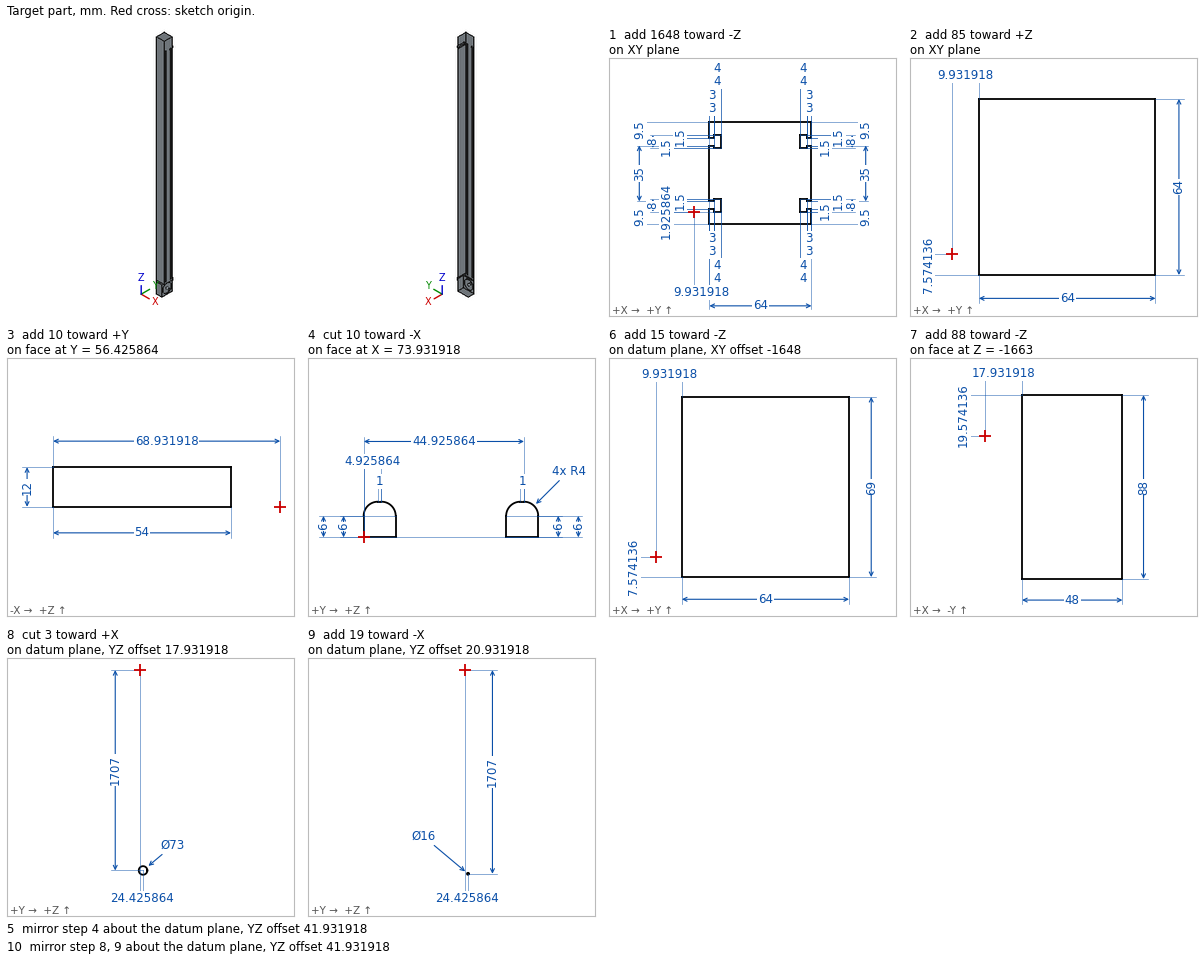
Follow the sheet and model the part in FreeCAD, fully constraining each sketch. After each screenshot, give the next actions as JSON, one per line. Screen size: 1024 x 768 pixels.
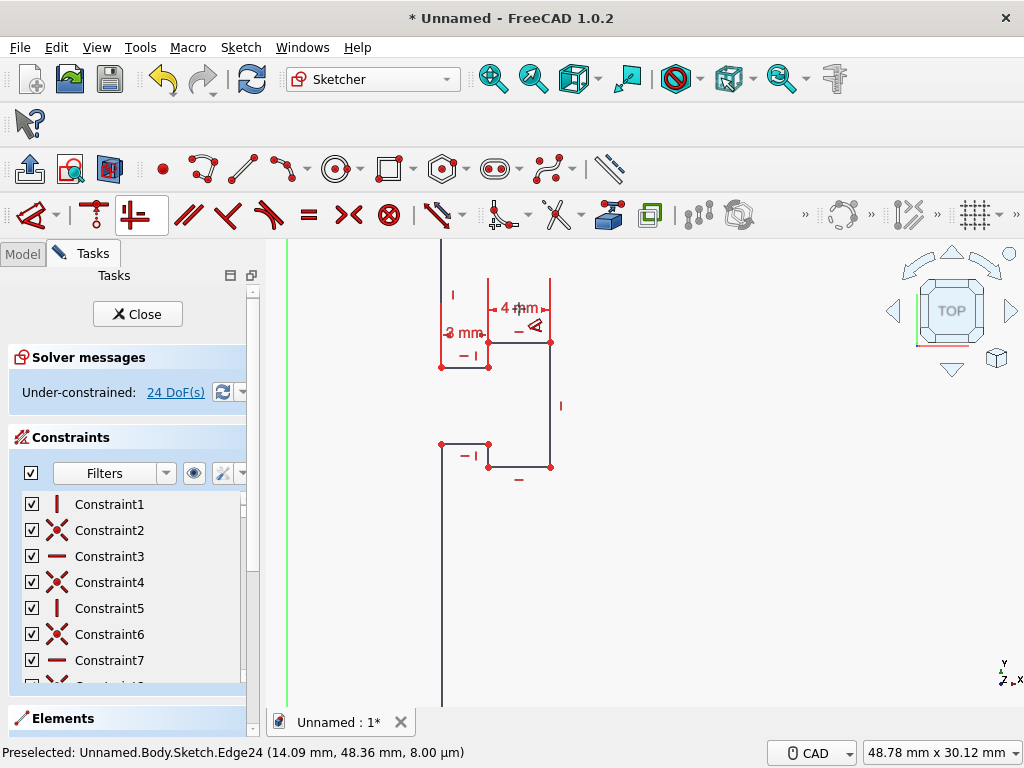
{"action": "left_click", "coordinate": [550, 380]}
{"action": "left_click", "coordinate": [516, 405]}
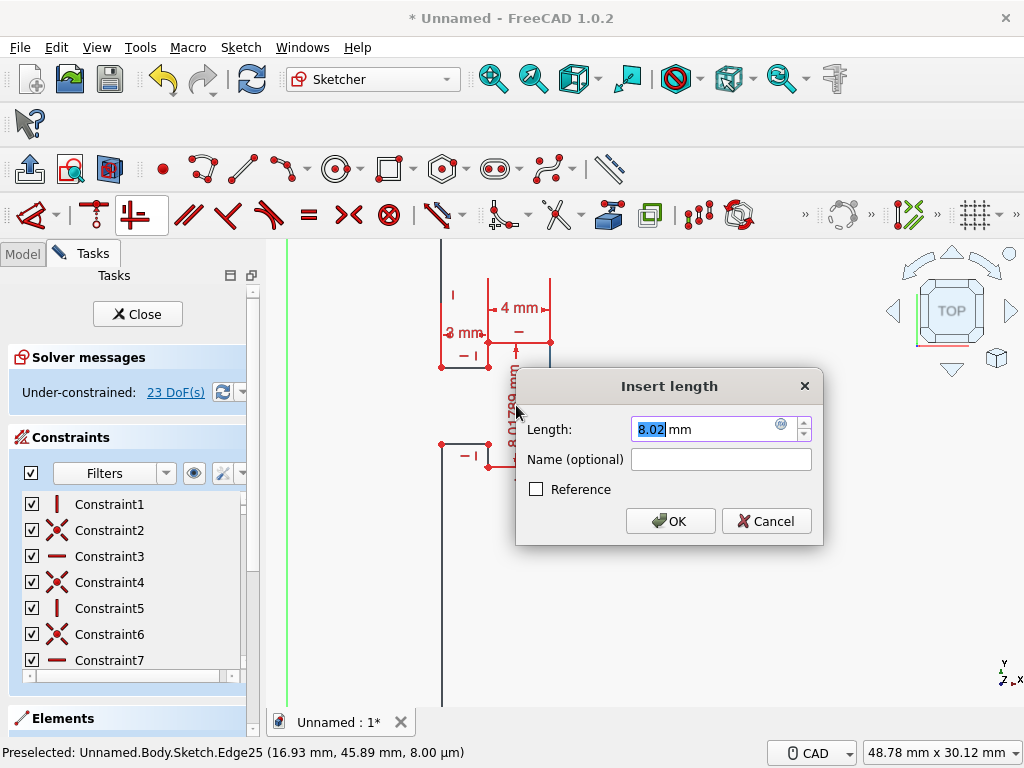
{"action": "type", "text": "8"}
{"action": "key", "text": "Return"}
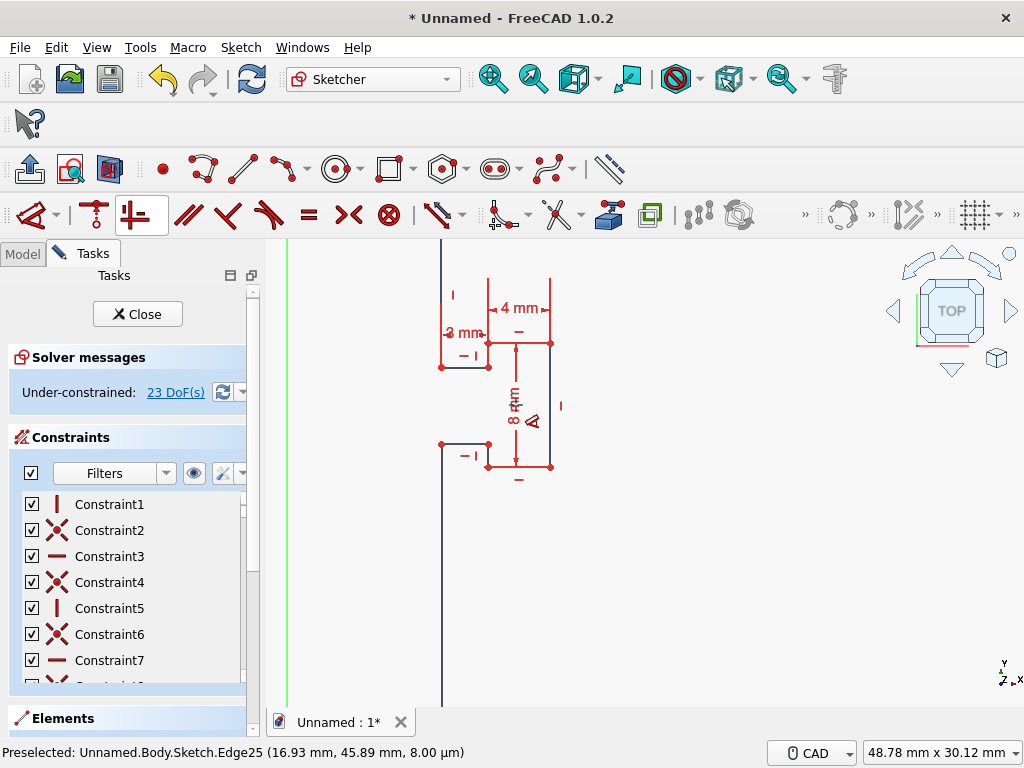
{"action": "left_click", "coordinate": [532, 467]}
{"action": "left_click", "coordinate": [519, 433]}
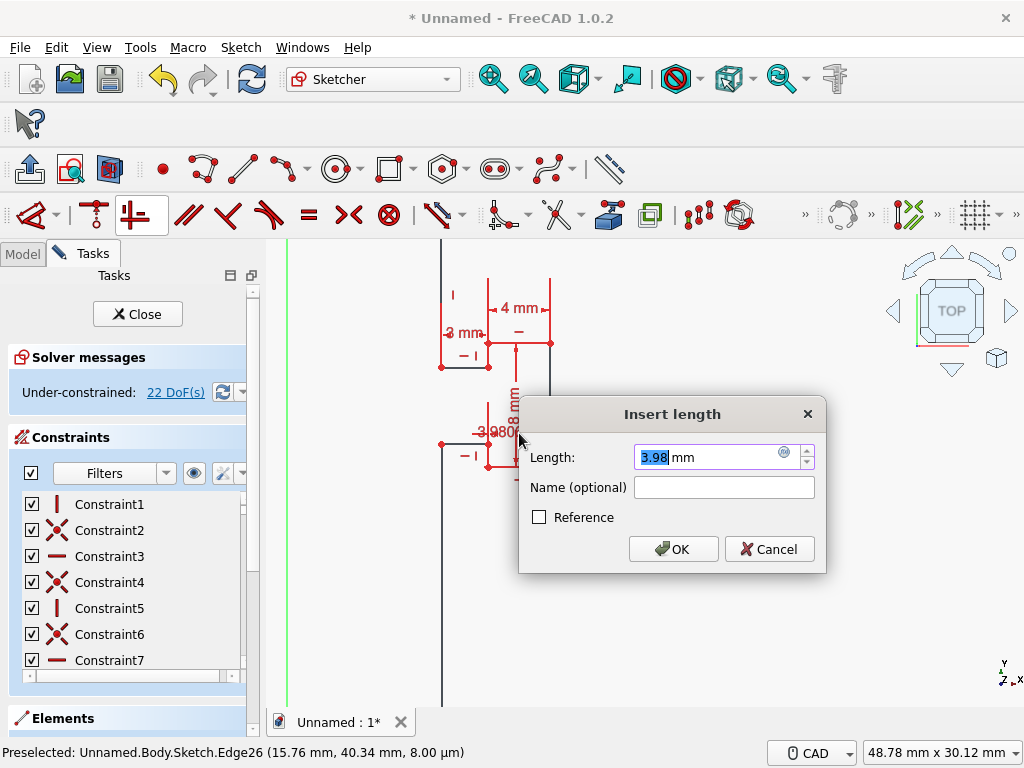
{"action": "type", "text": "4"}
{"action": "key", "text": "Return"}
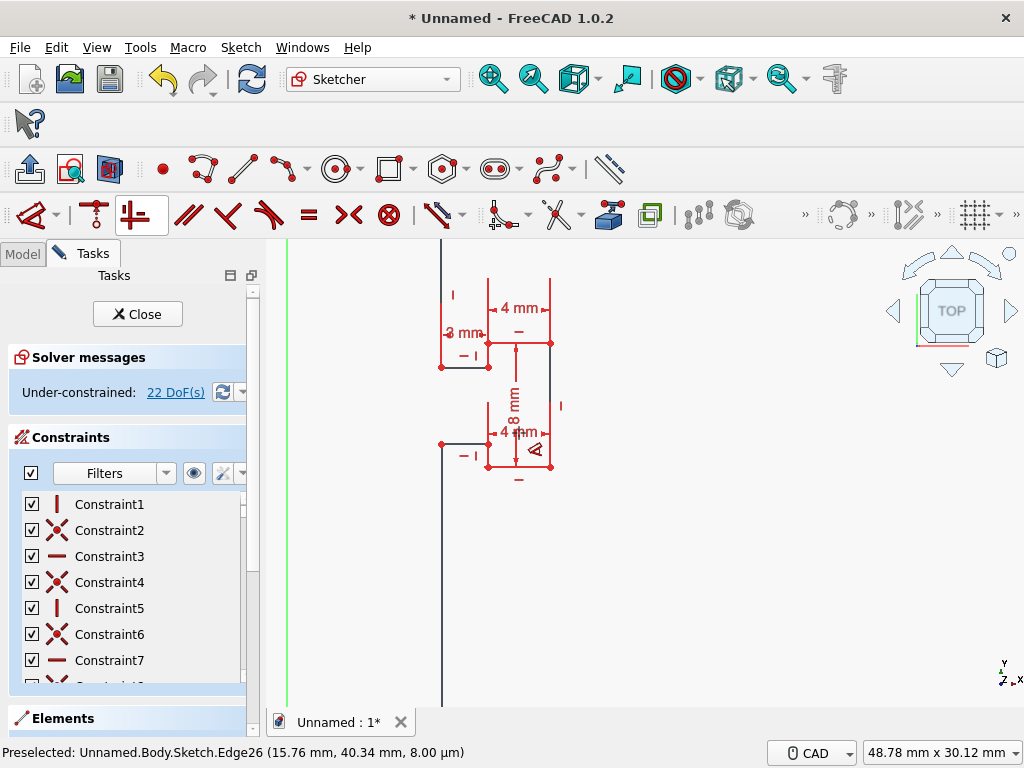
{"action": "left_click", "coordinate": [474, 444]}
{"action": "left_click", "coordinate": [465, 478]}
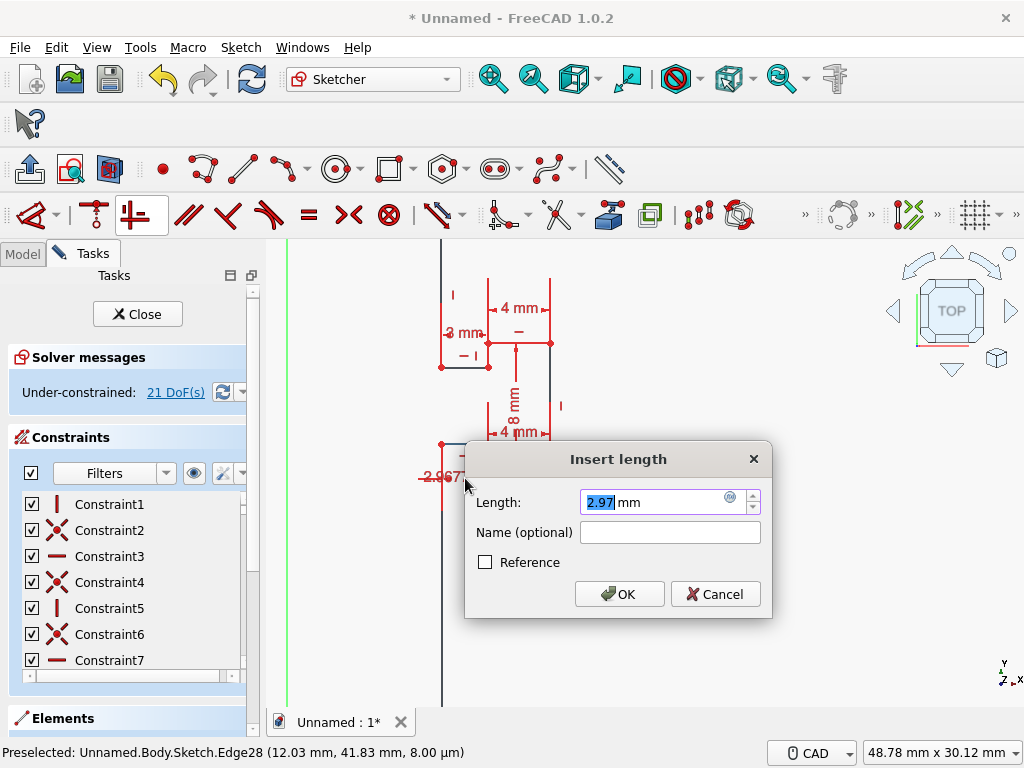
{"action": "type", "text": "3"}
{"action": "key", "text": "Return"}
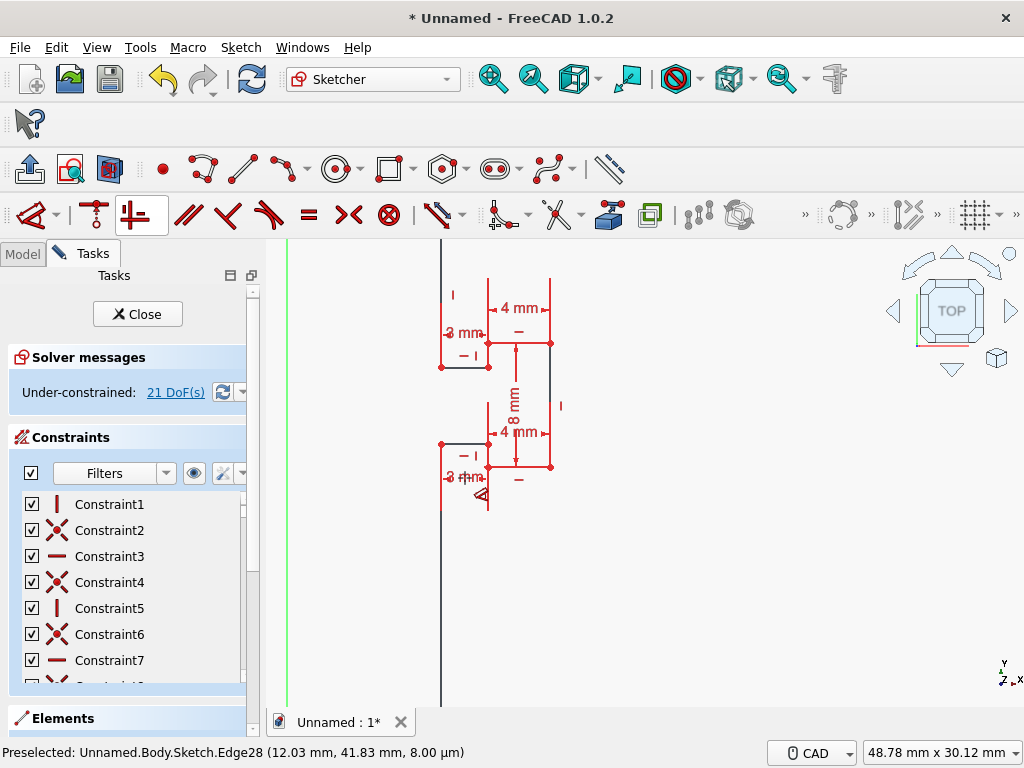
{"action": "scroll", "coordinate": [454, 369], "scroll_direction": "down", "scroll_amount": 6}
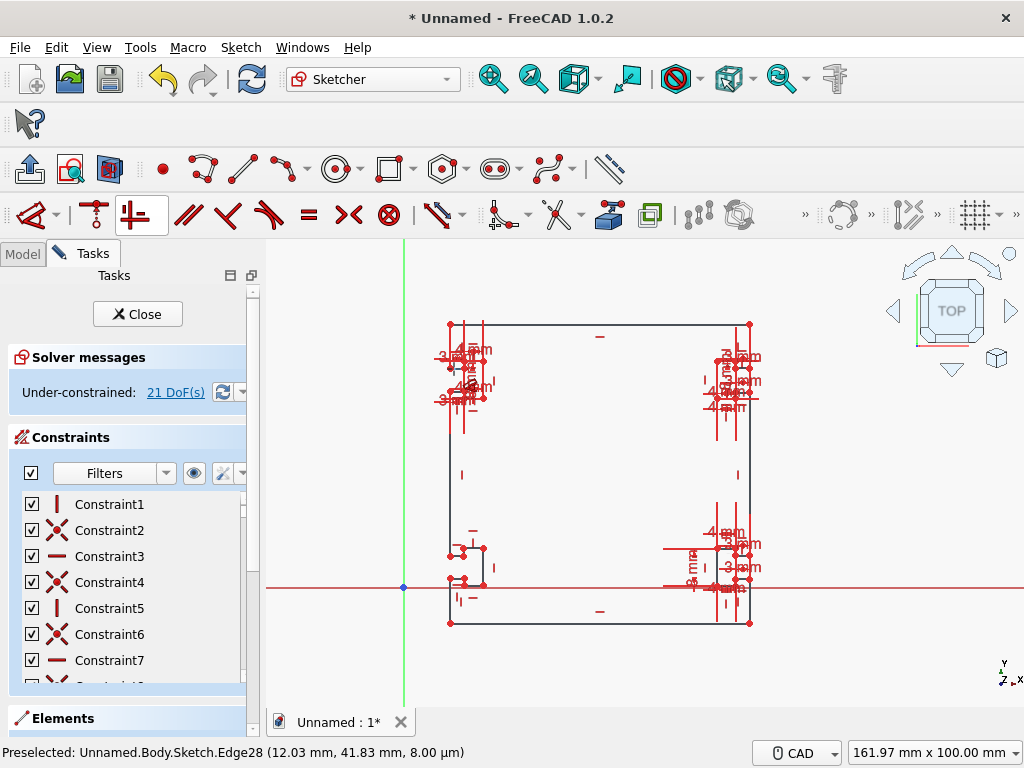
{"action": "scroll", "coordinate": [454, 556], "scroll_direction": "up", "scroll_amount": 7}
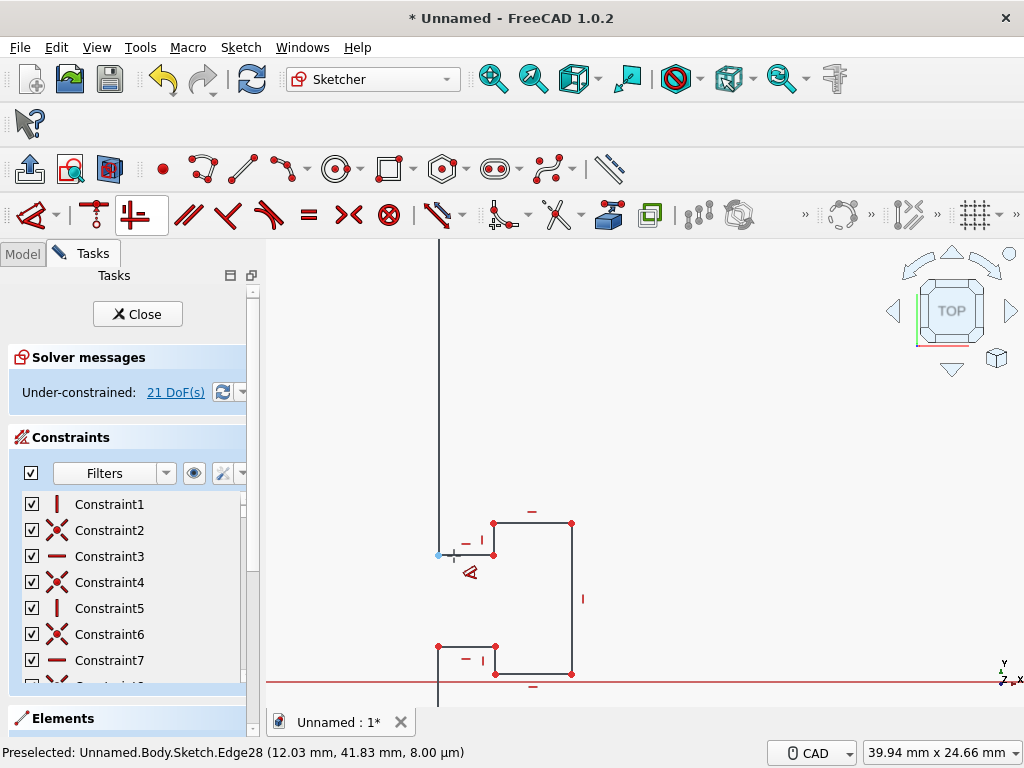
{"action": "left_click", "coordinate": [455, 555]}
{"action": "left_click", "coordinate": [466, 589]}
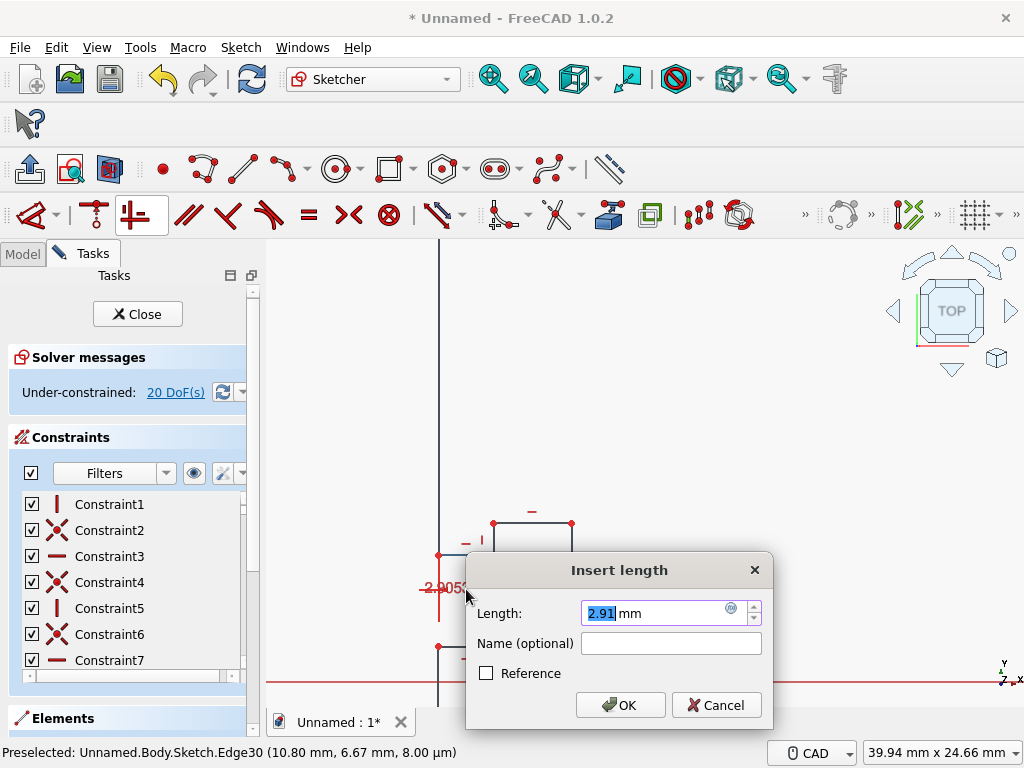
{"action": "type", "text": "3"}
{"action": "key", "text": "Return"}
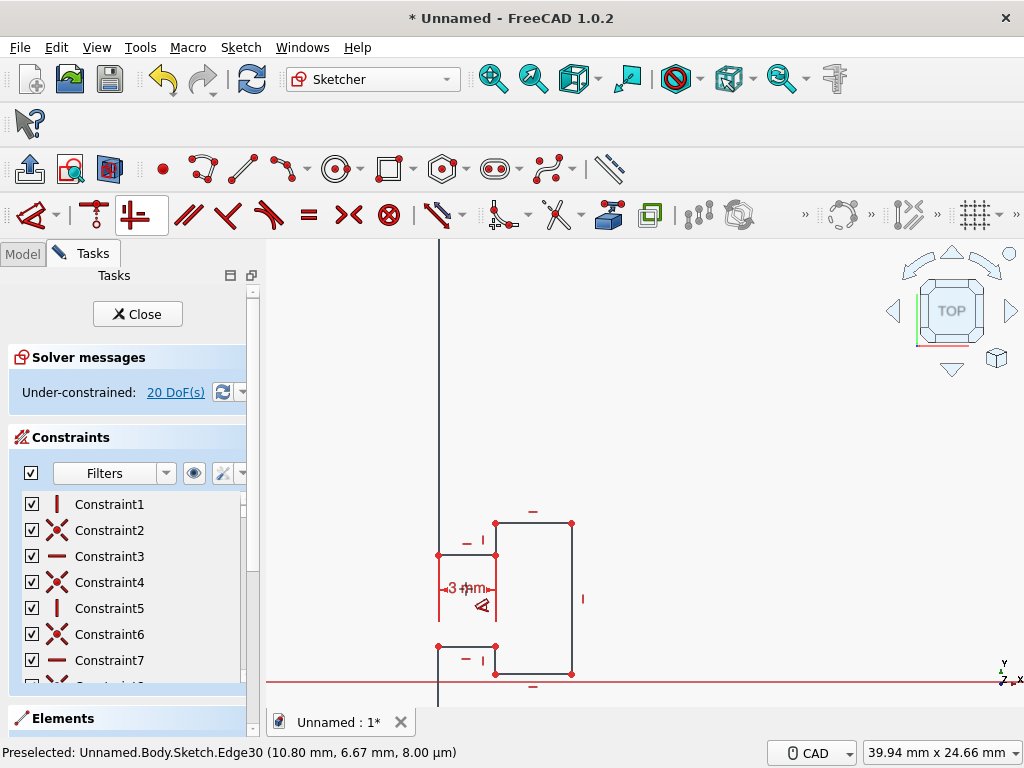
{"action": "left_click", "coordinate": [518, 523]}
{"action": "left_click", "coordinate": [534, 557]}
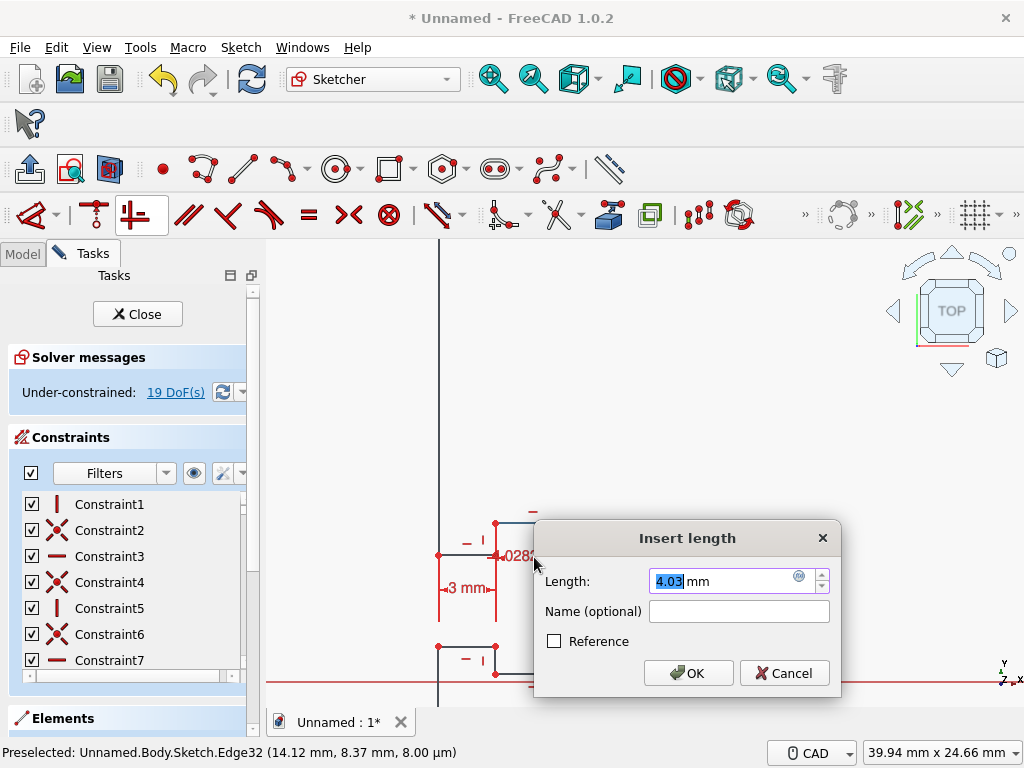
{"action": "type", "text": "4"}
{"action": "key", "text": "Return"}